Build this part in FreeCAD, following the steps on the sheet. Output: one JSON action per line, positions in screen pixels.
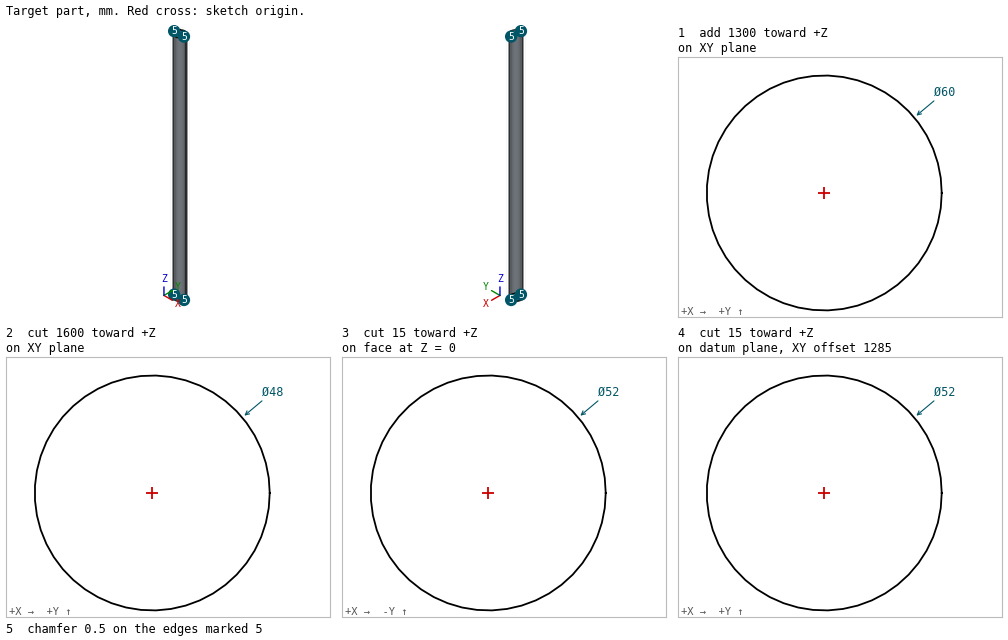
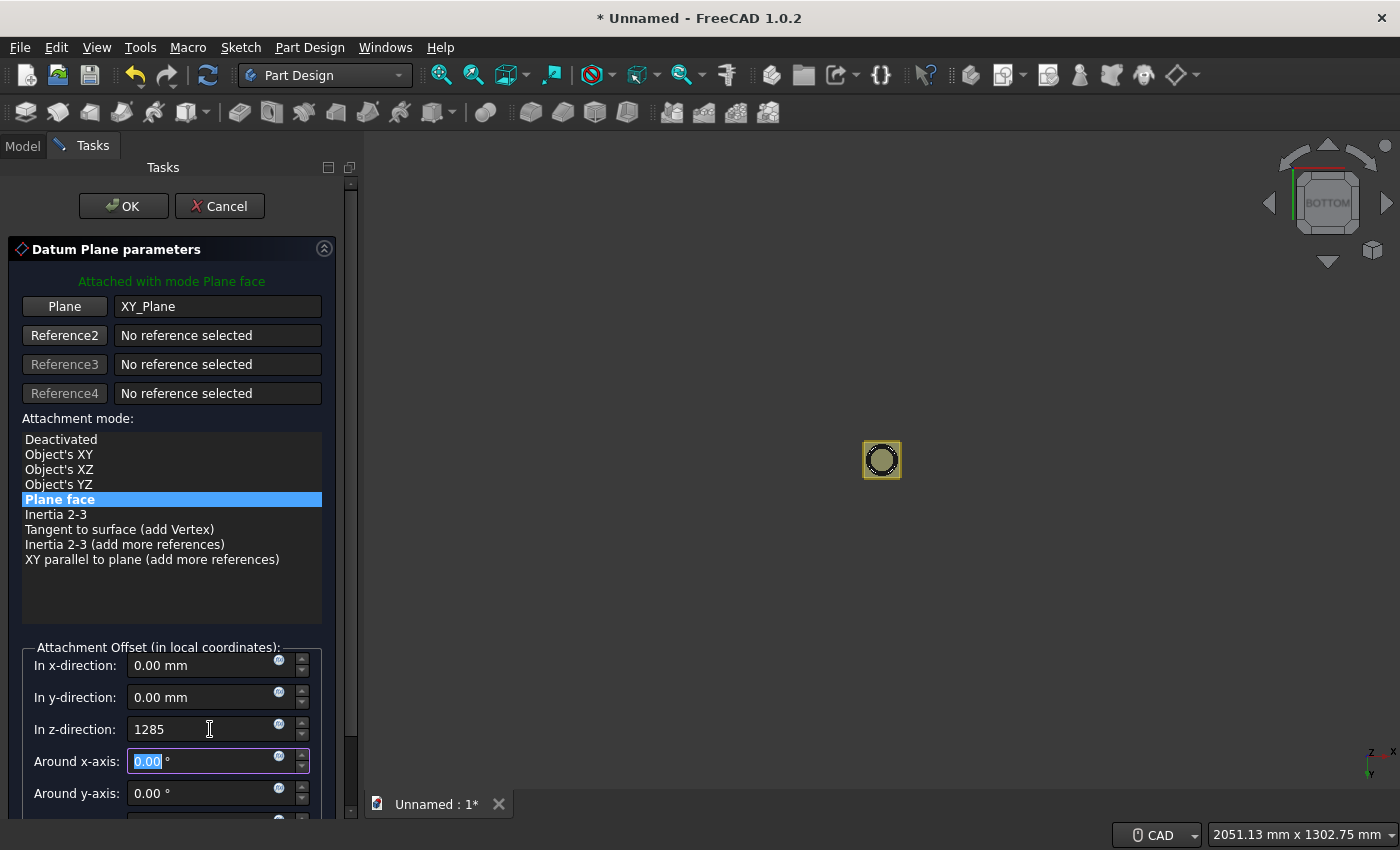
{"action": "left_click", "coordinate": [124, 206]}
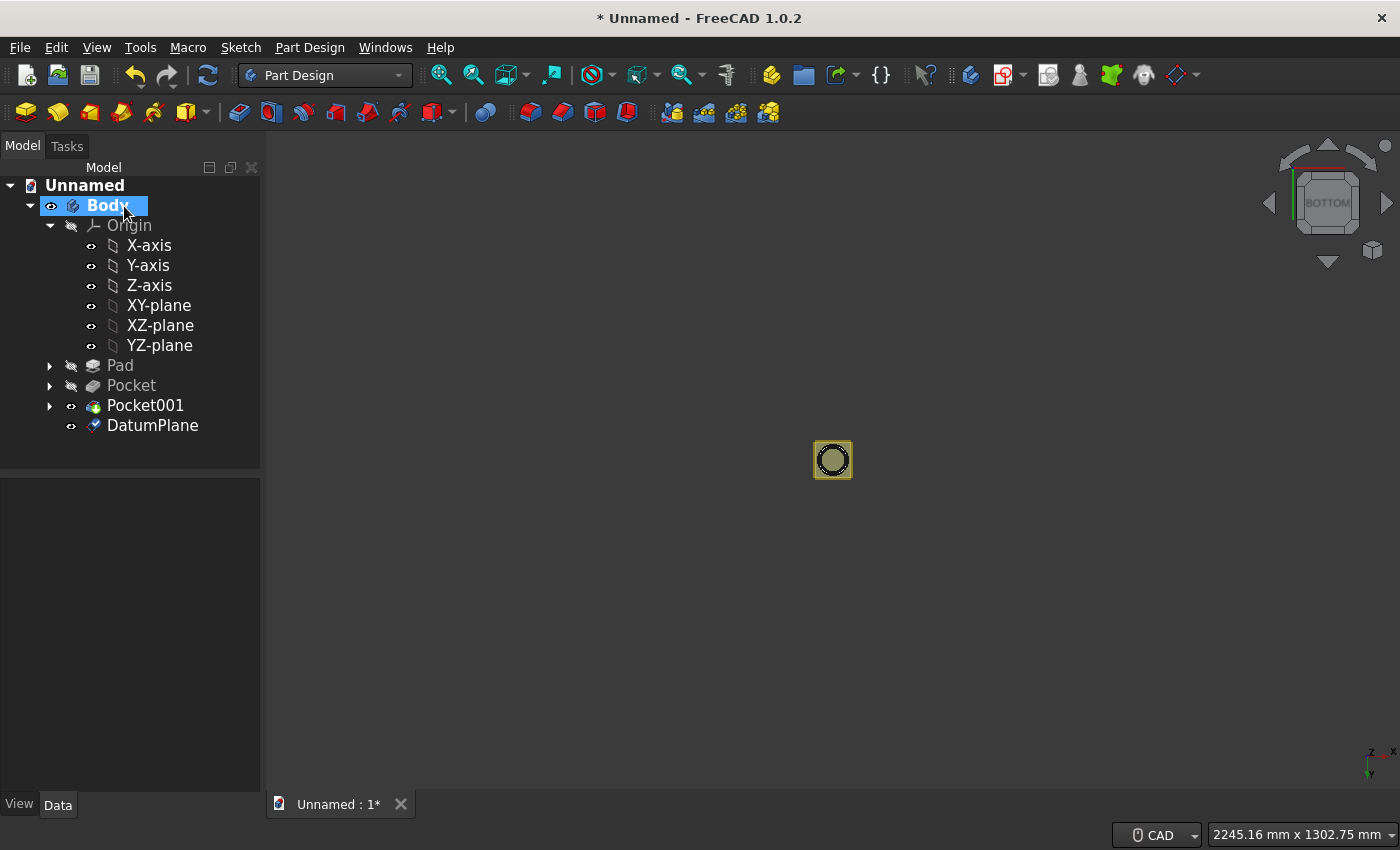
{"action": "left_click", "coordinate": [116, 426]}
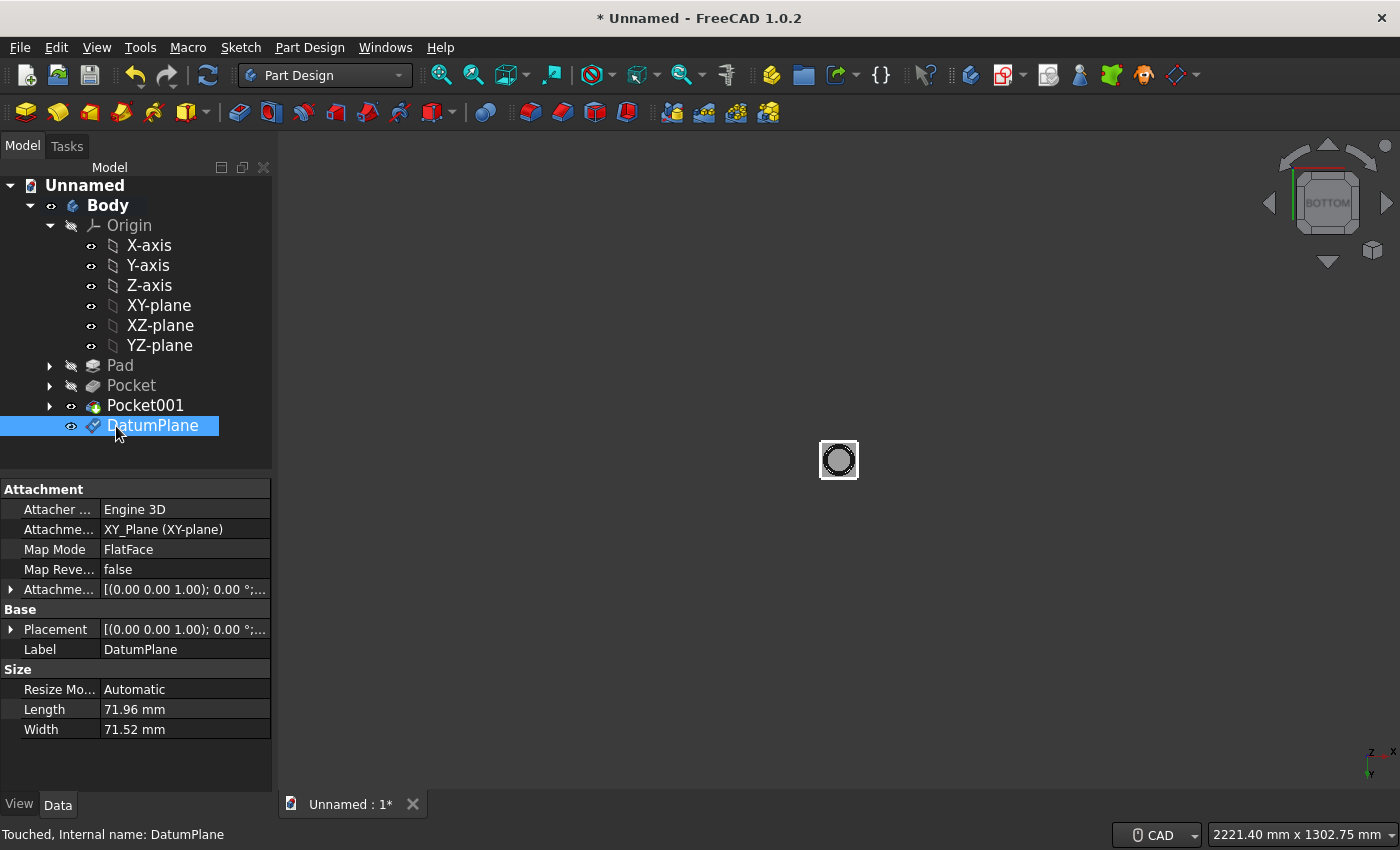
{"action": "left_click", "coordinate": [1004, 76]}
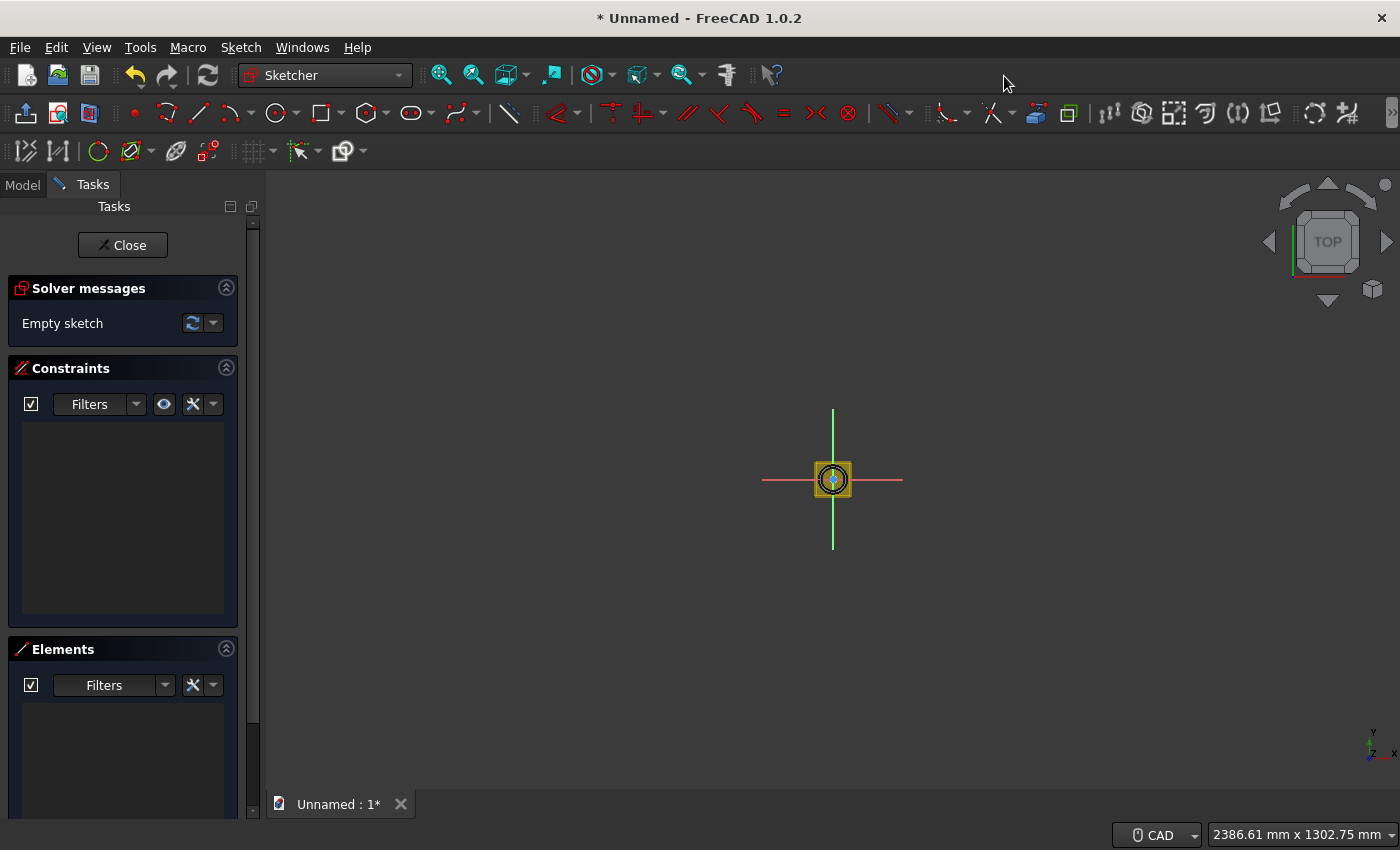
{"action": "left_click", "coordinate": [90, 114]}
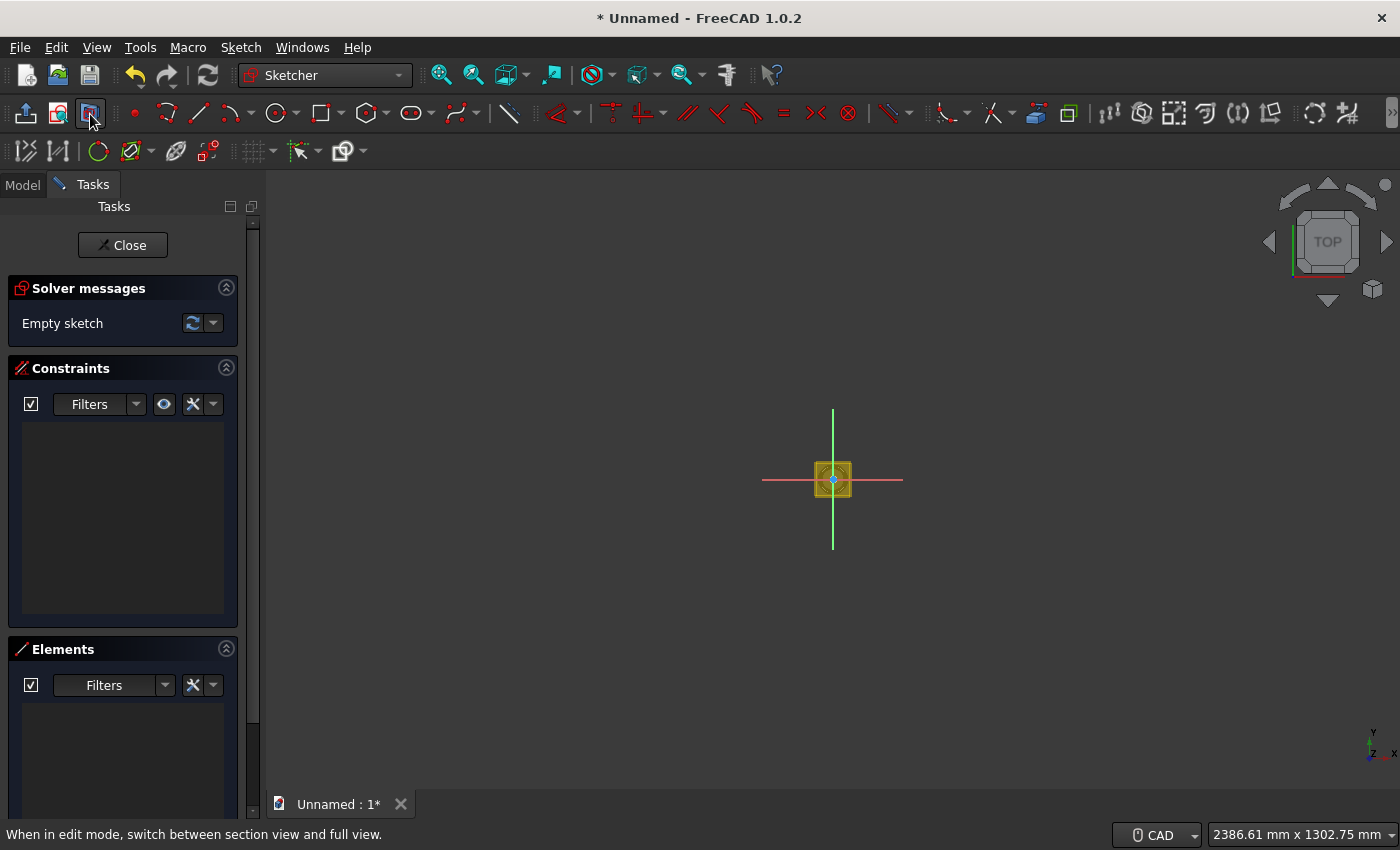
{"action": "scroll", "coordinate": [837, 480], "scroll_direction": "up", "scroll_amount": 14}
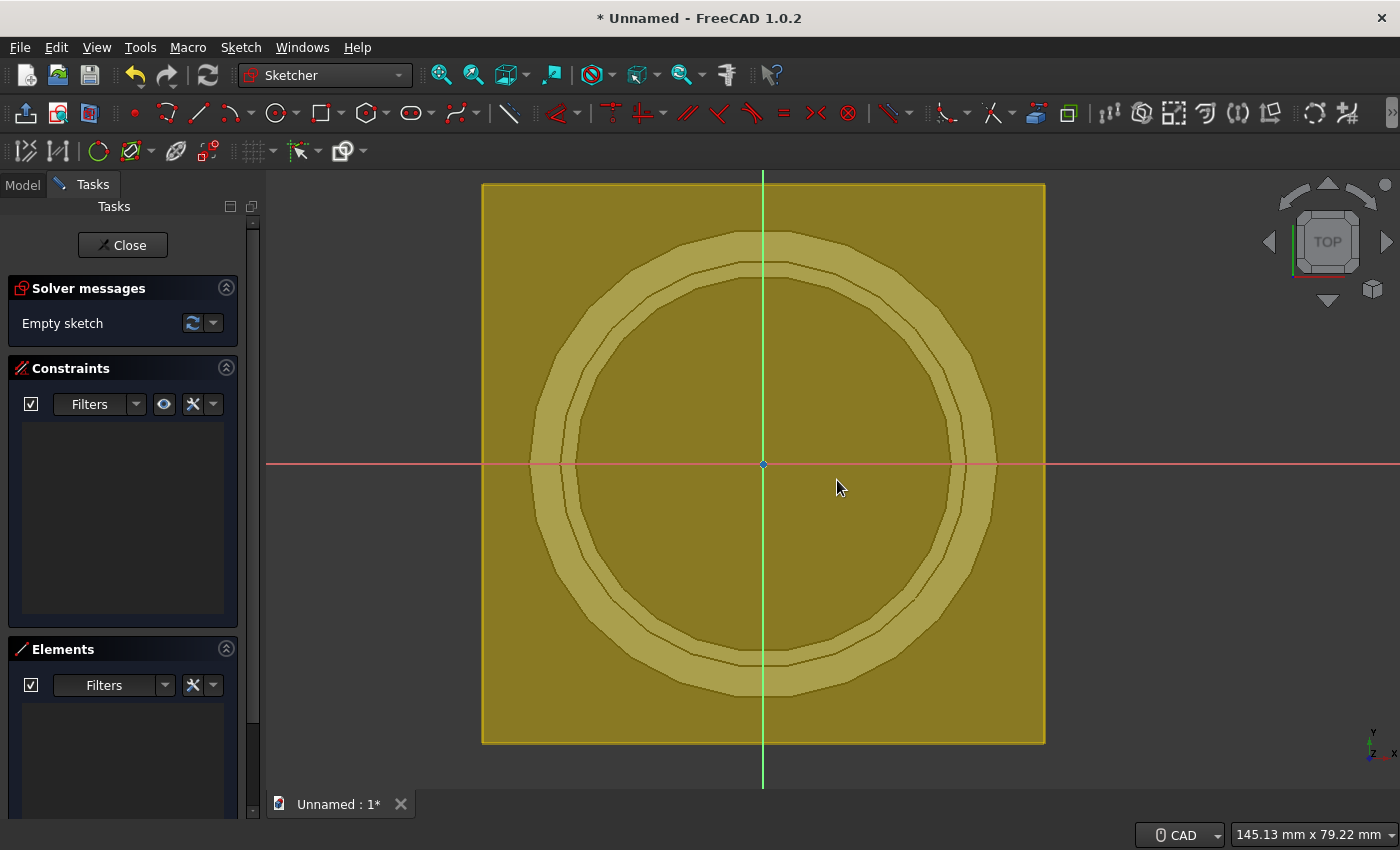
{"action": "left_click", "coordinate": [276, 114]}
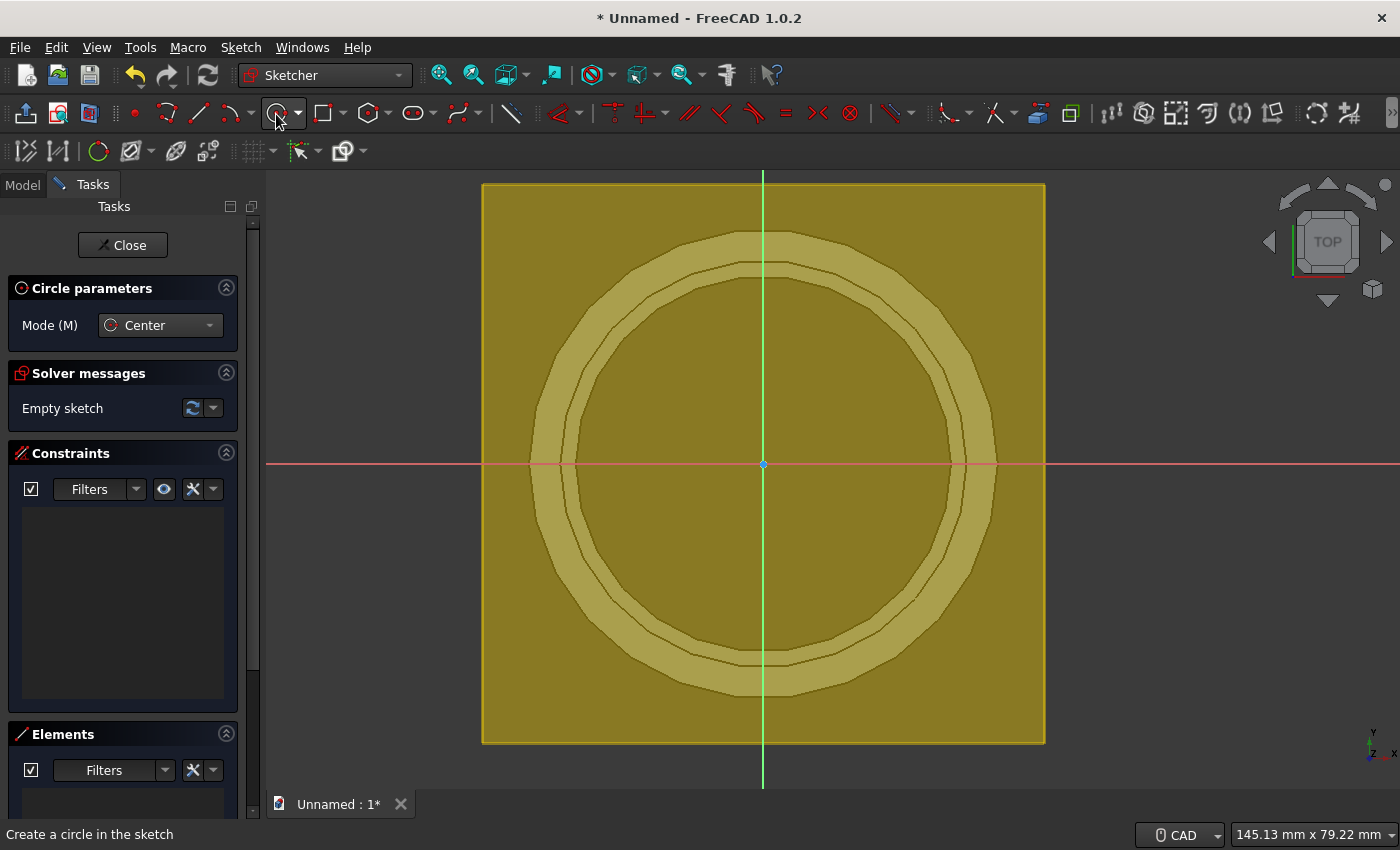
{"action": "left_click", "coordinate": [763, 464]}
{"action": "mouse_move", "coordinate": [907, 320]}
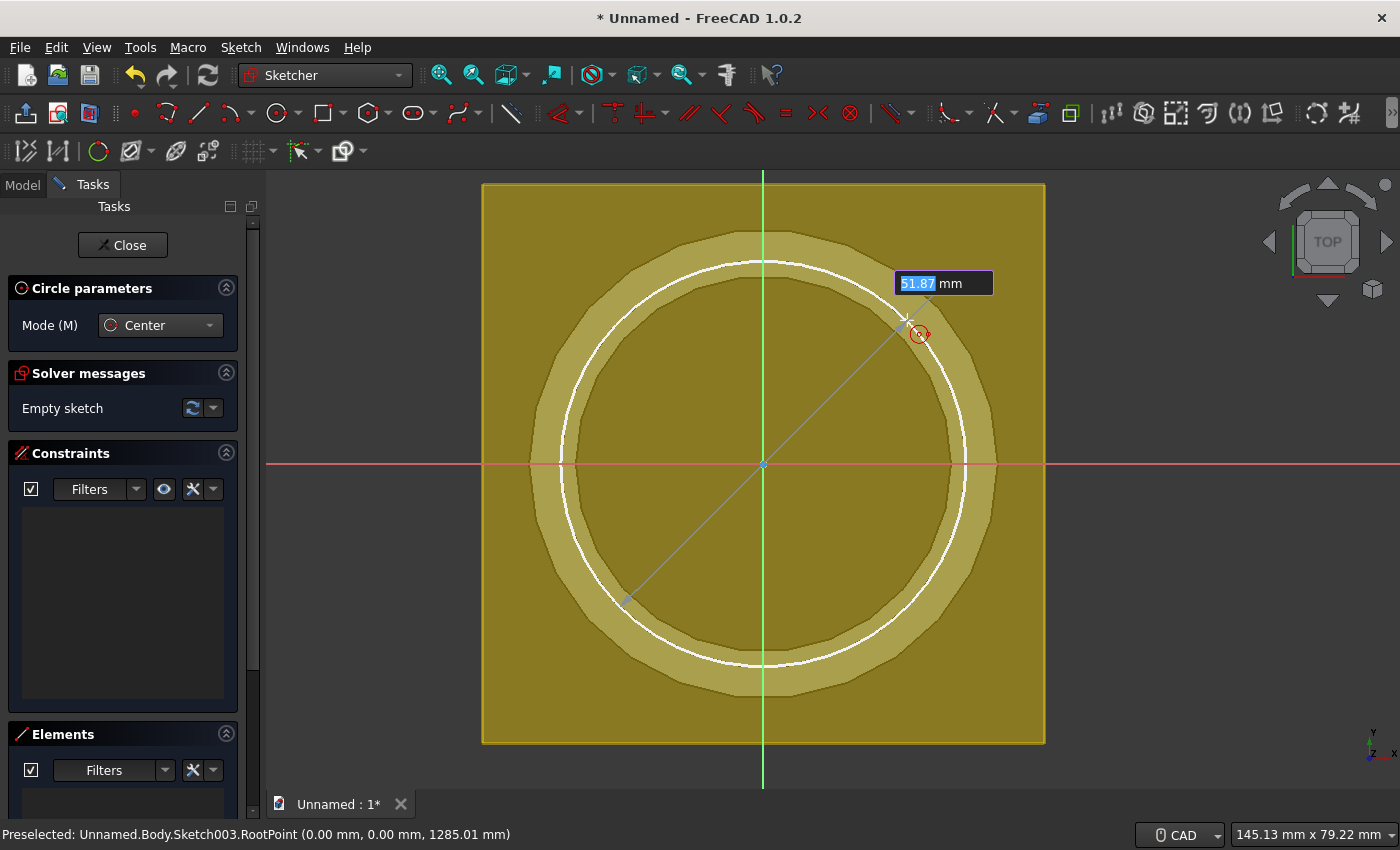
{"action": "type", "text": "52"}
{"action": "key", "text": "Return"}
{"action": "key", "text": "Escape"}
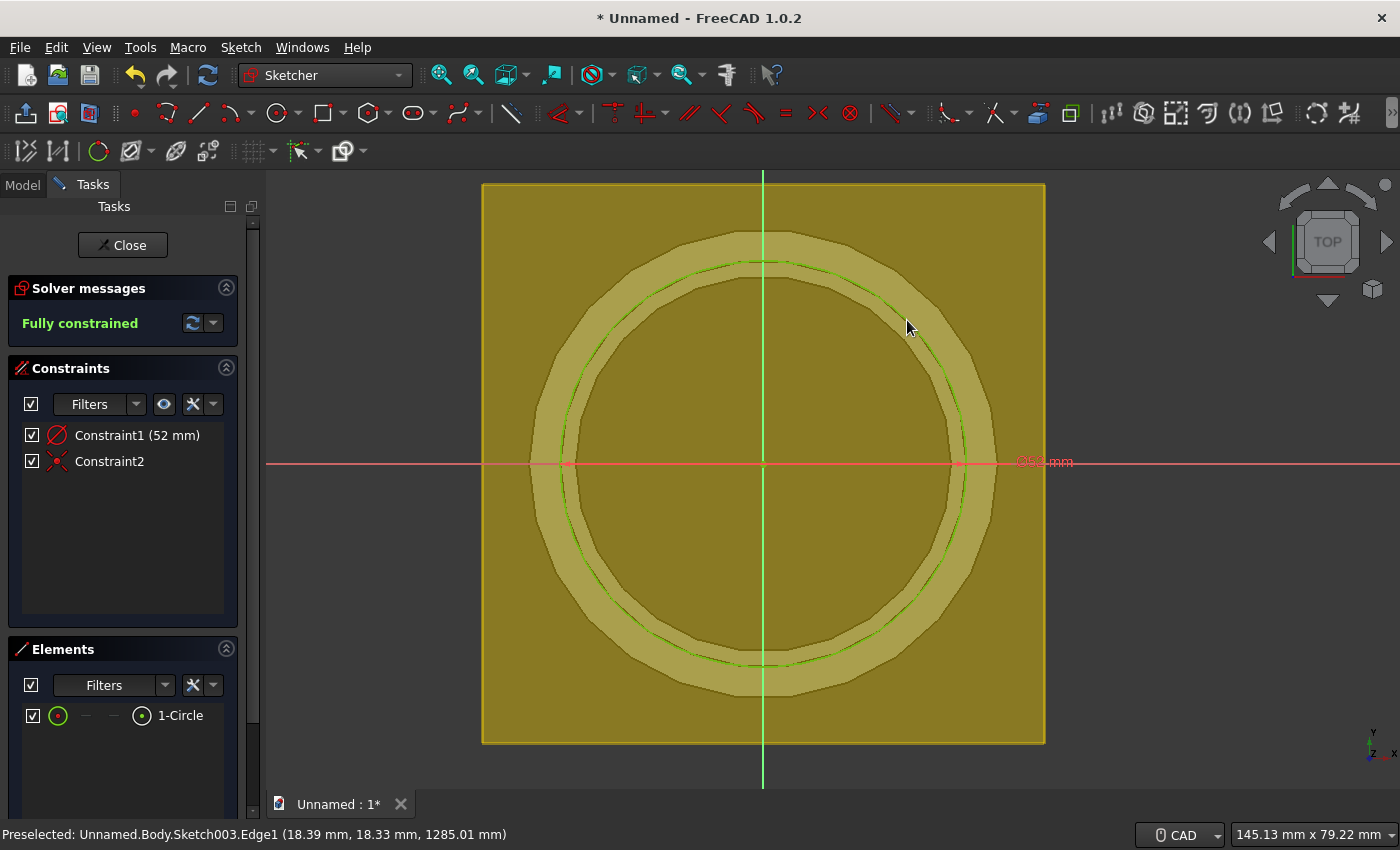
{"action": "left_click", "coordinate": [123, 245]}